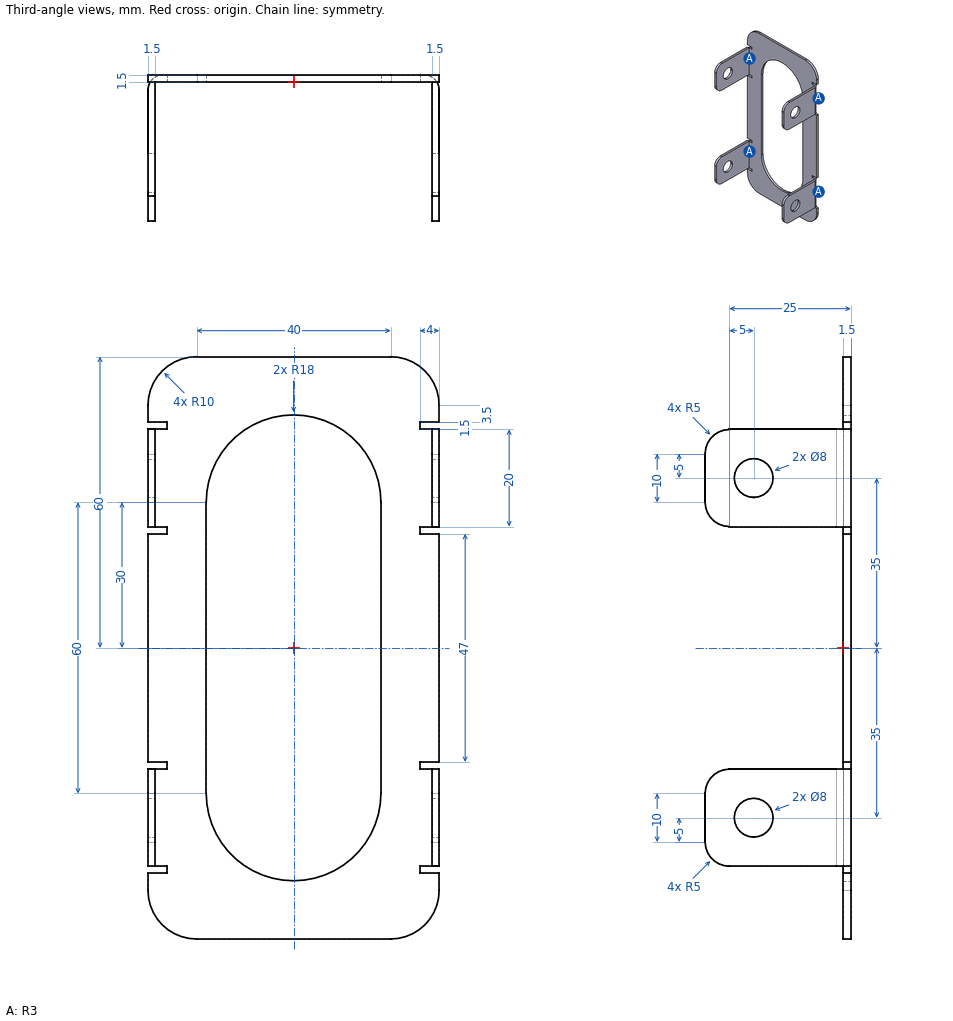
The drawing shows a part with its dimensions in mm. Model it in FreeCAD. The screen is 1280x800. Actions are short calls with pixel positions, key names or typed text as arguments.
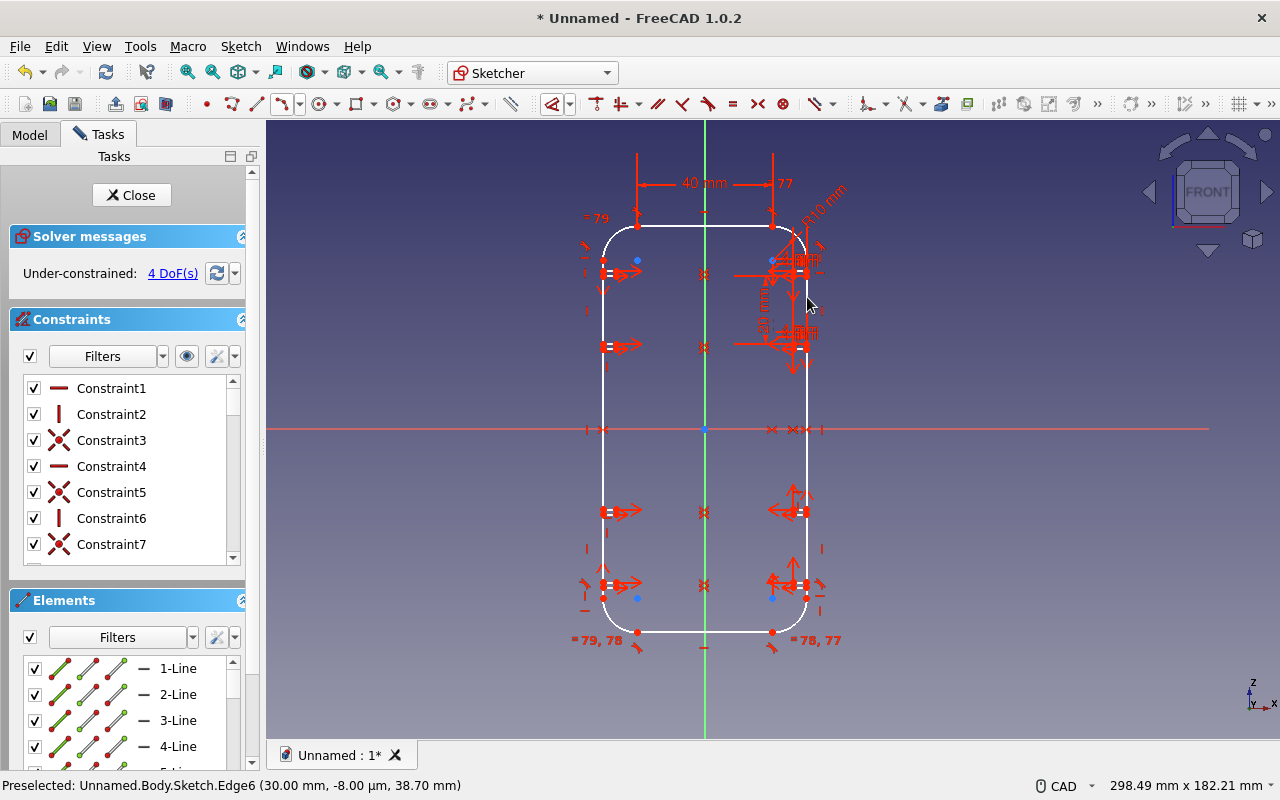
click(807, 397)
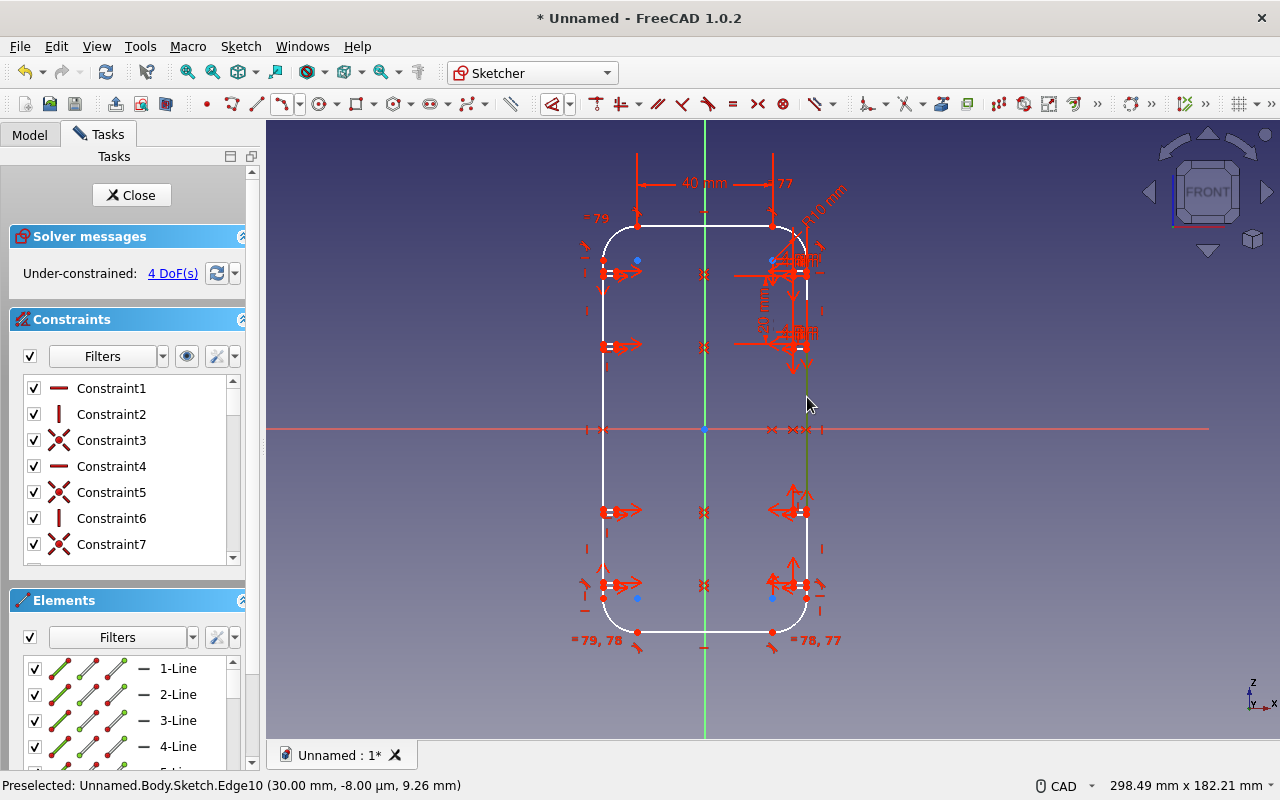
click(570, 104)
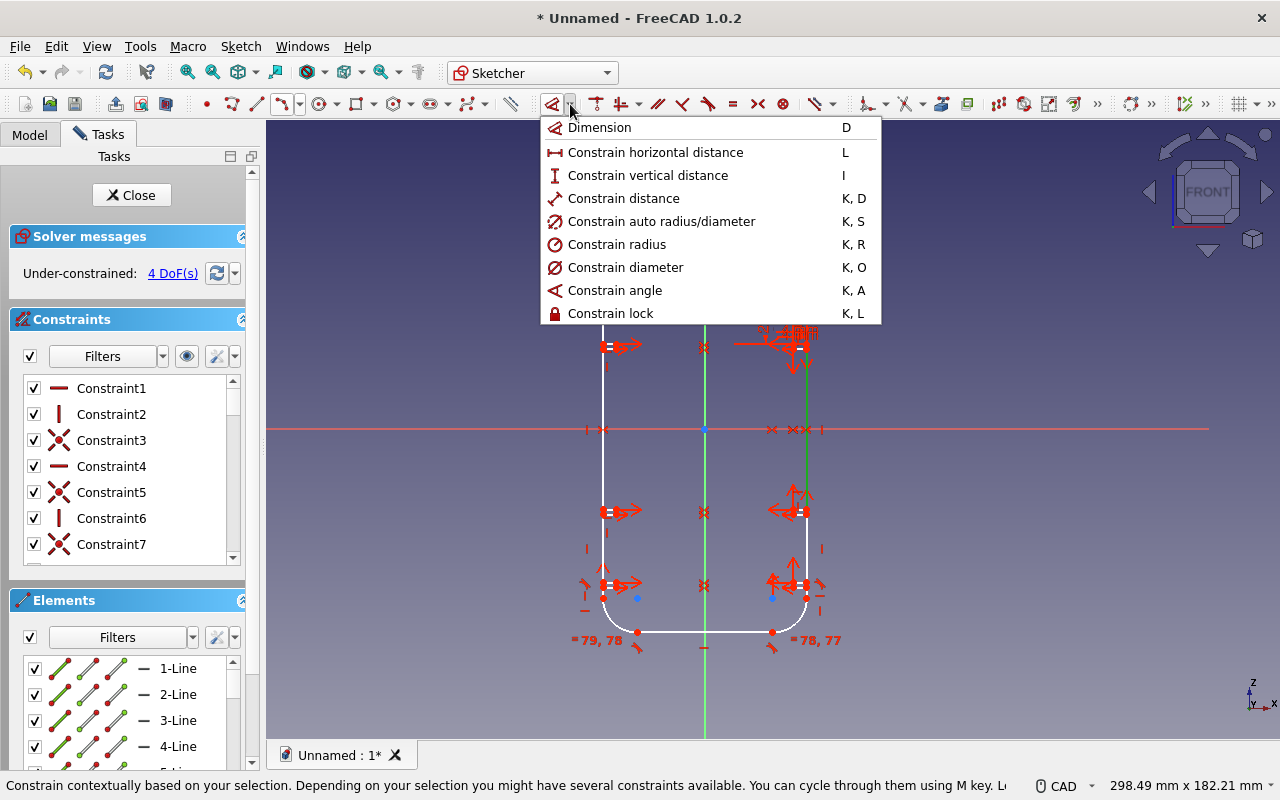
click(711, 176)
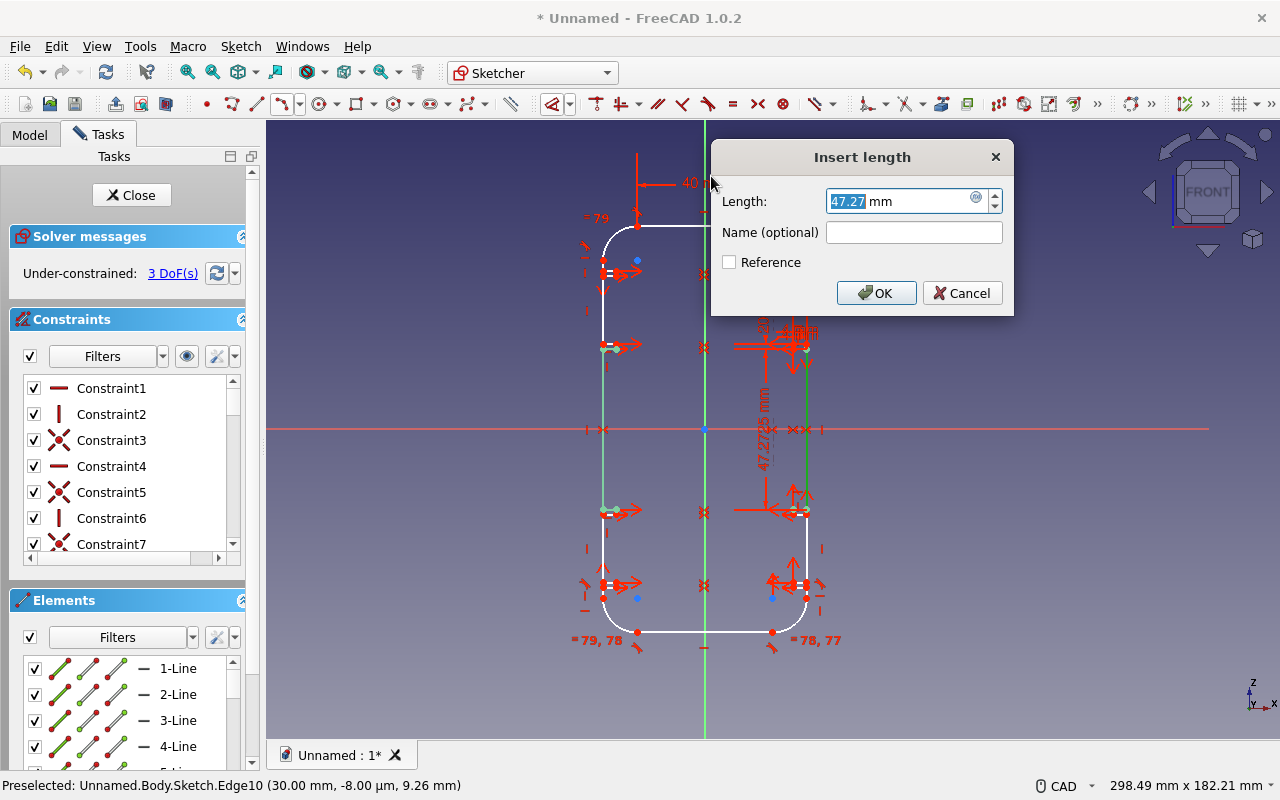
text(47)
key(Return)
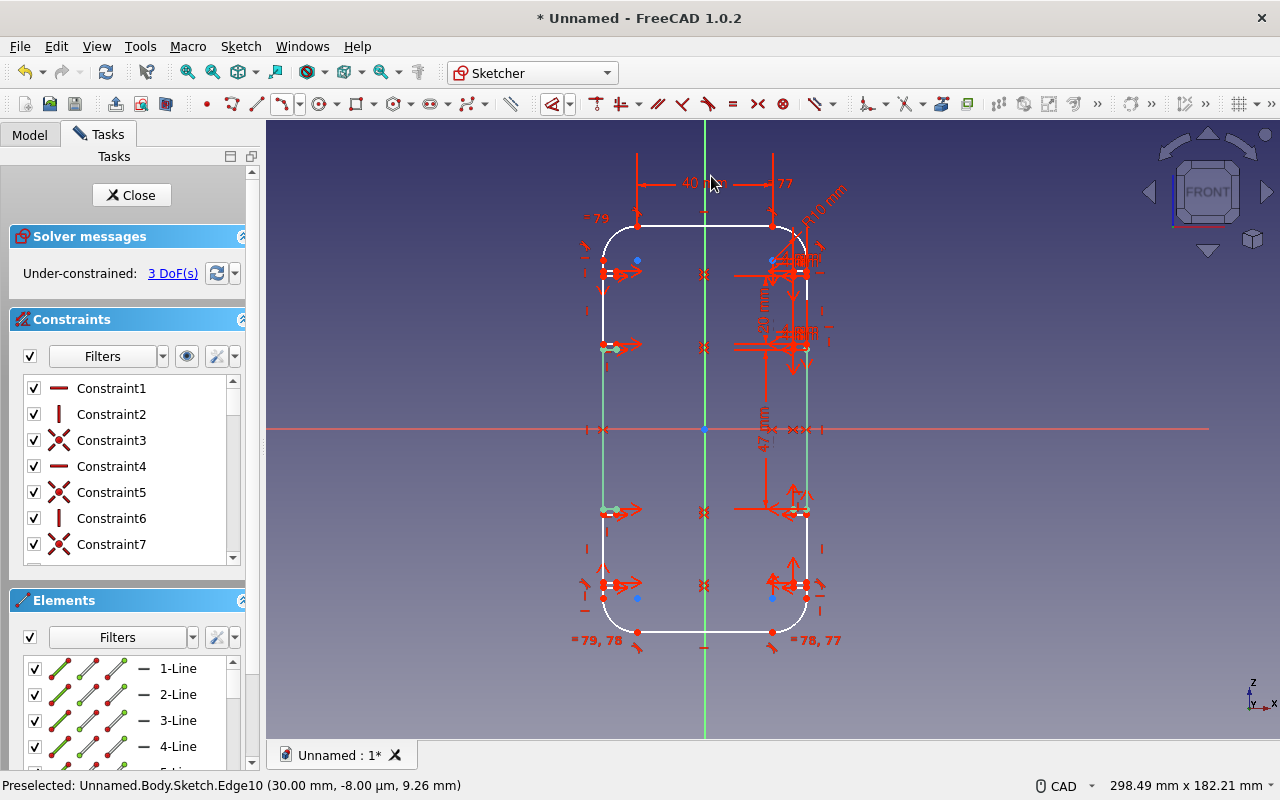
scroll(807, 266, up, 7)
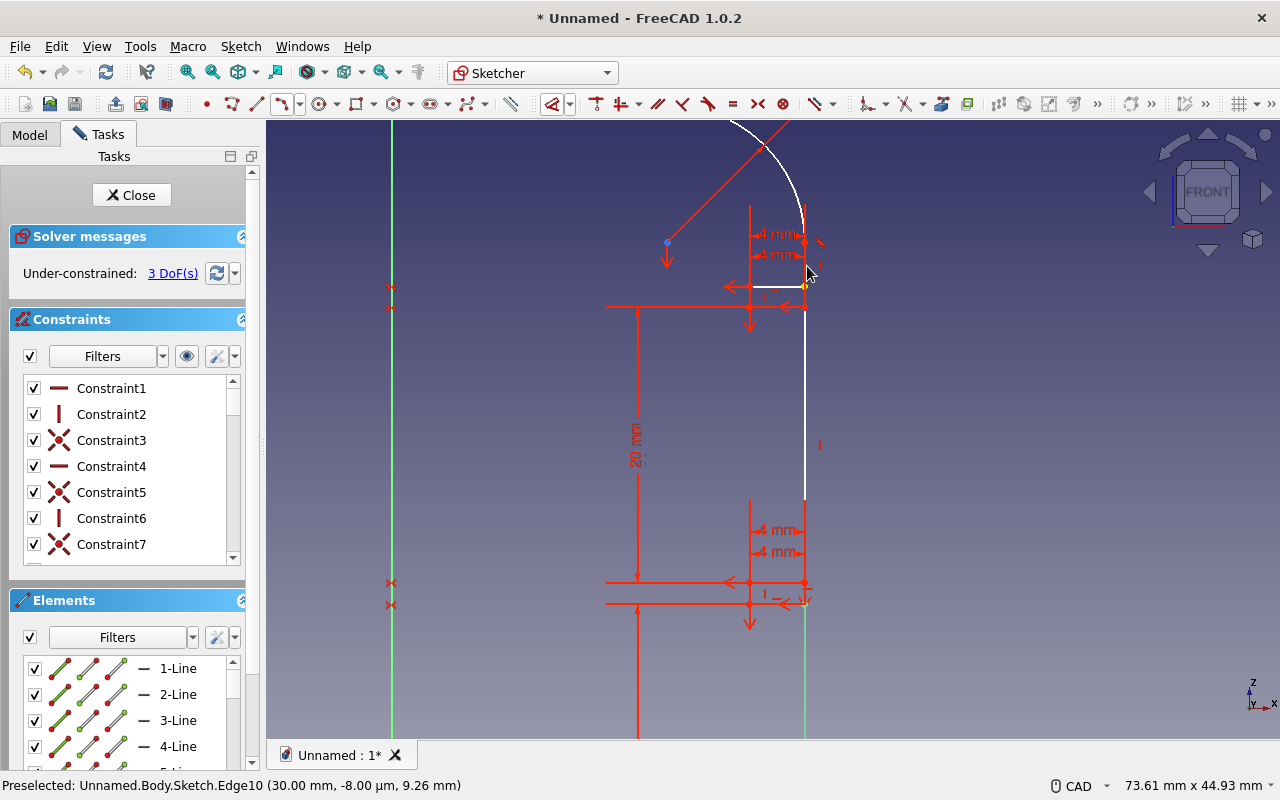
click(805, 265)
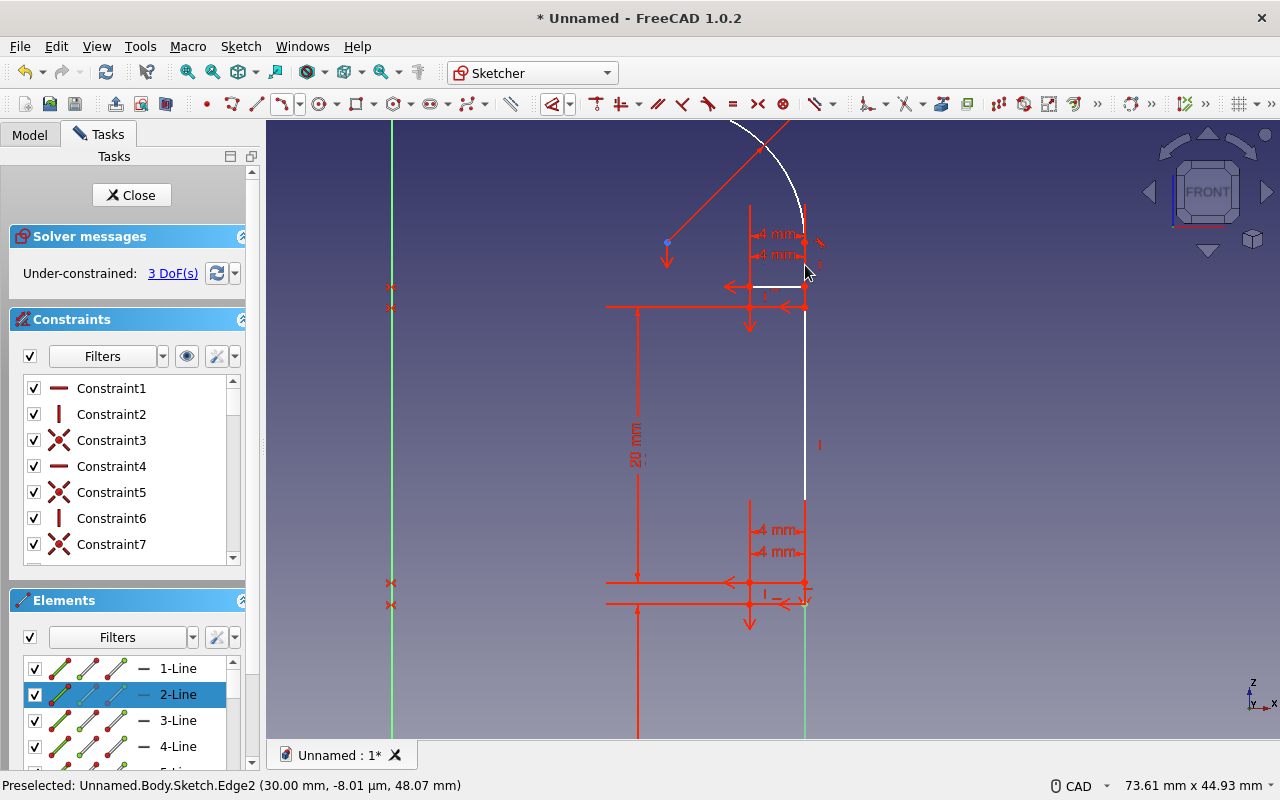
click(570, 104)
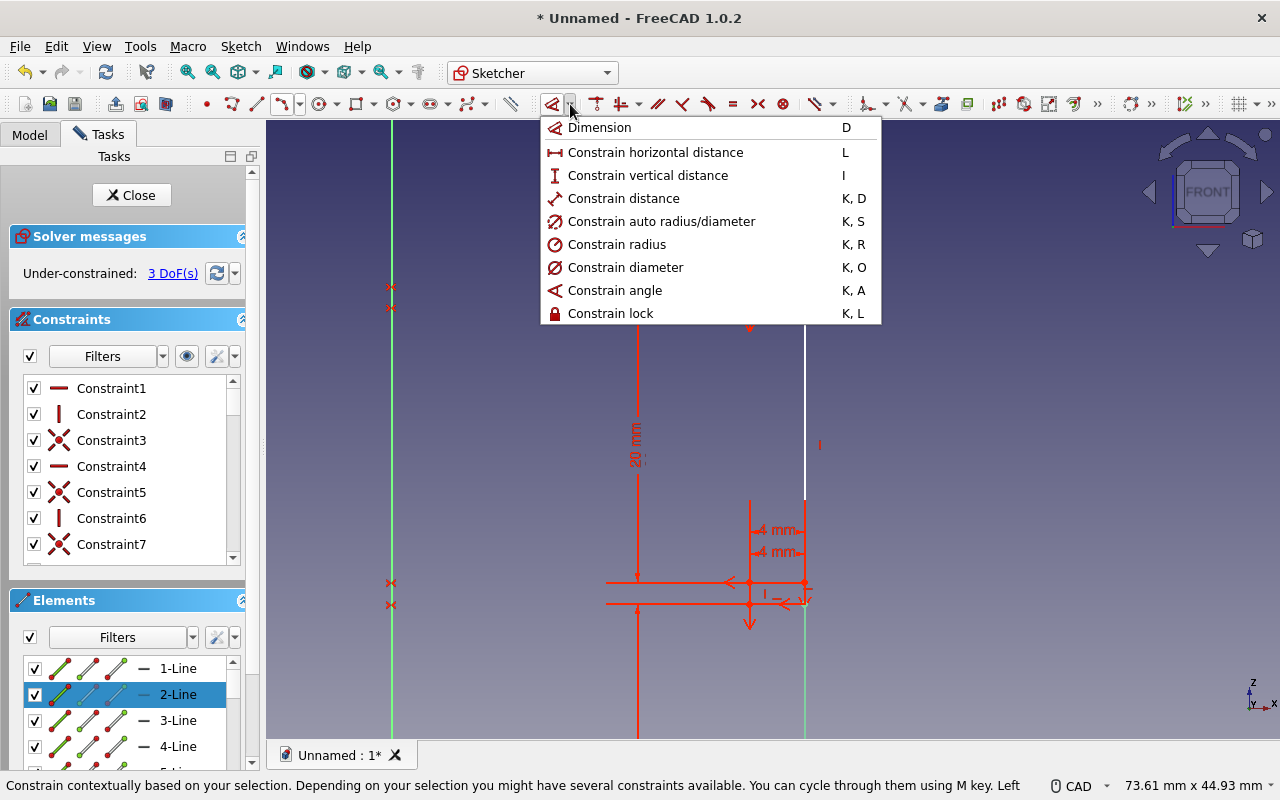
click(711, 176)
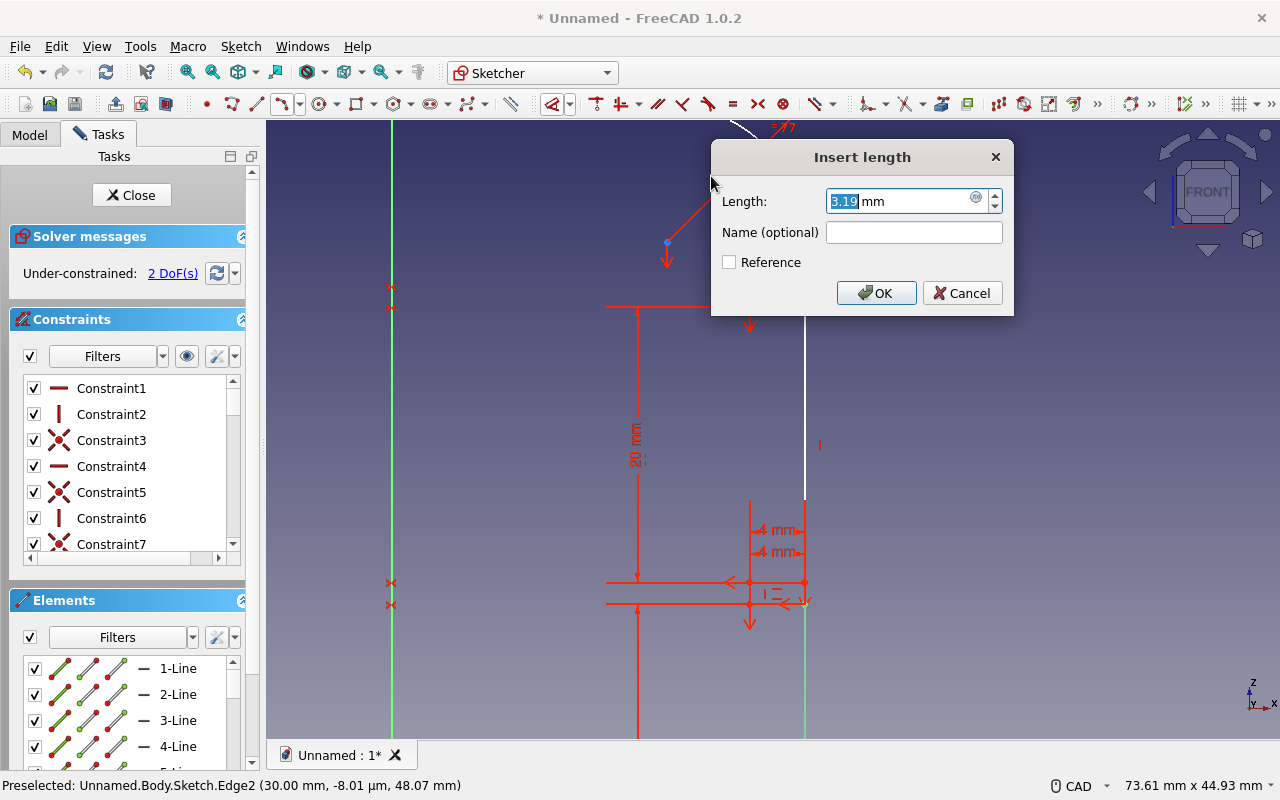
text(3.5)
key(Return)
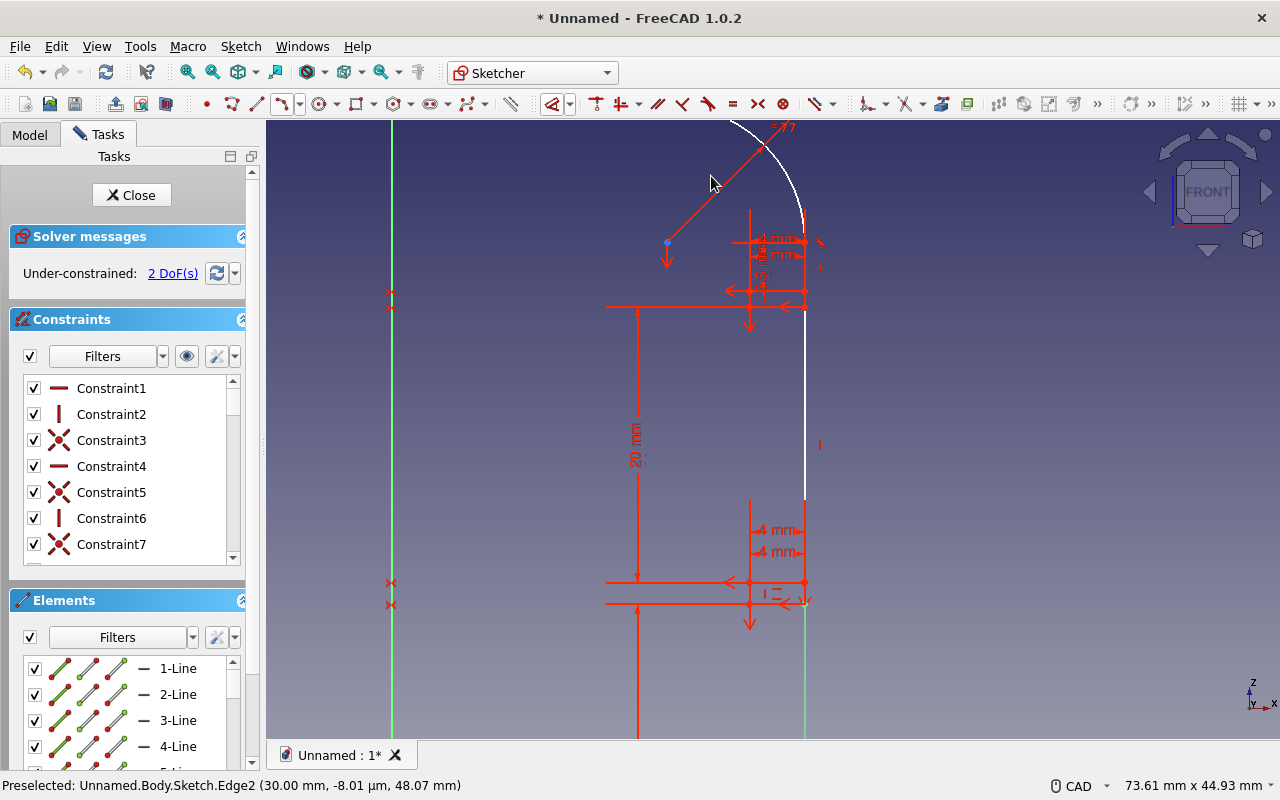
scroll(750, 299, up, 4)